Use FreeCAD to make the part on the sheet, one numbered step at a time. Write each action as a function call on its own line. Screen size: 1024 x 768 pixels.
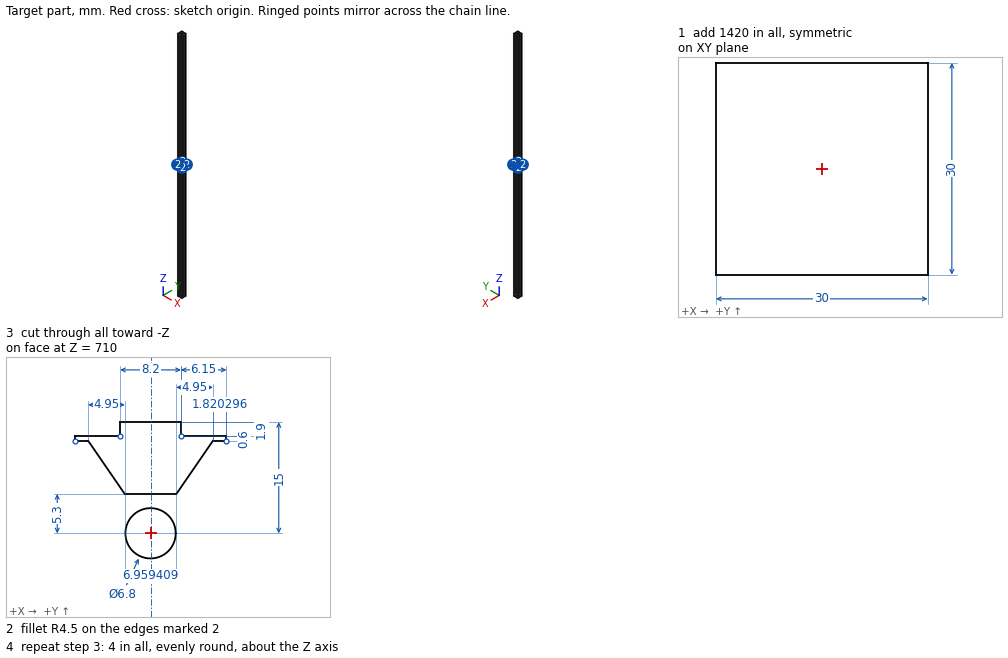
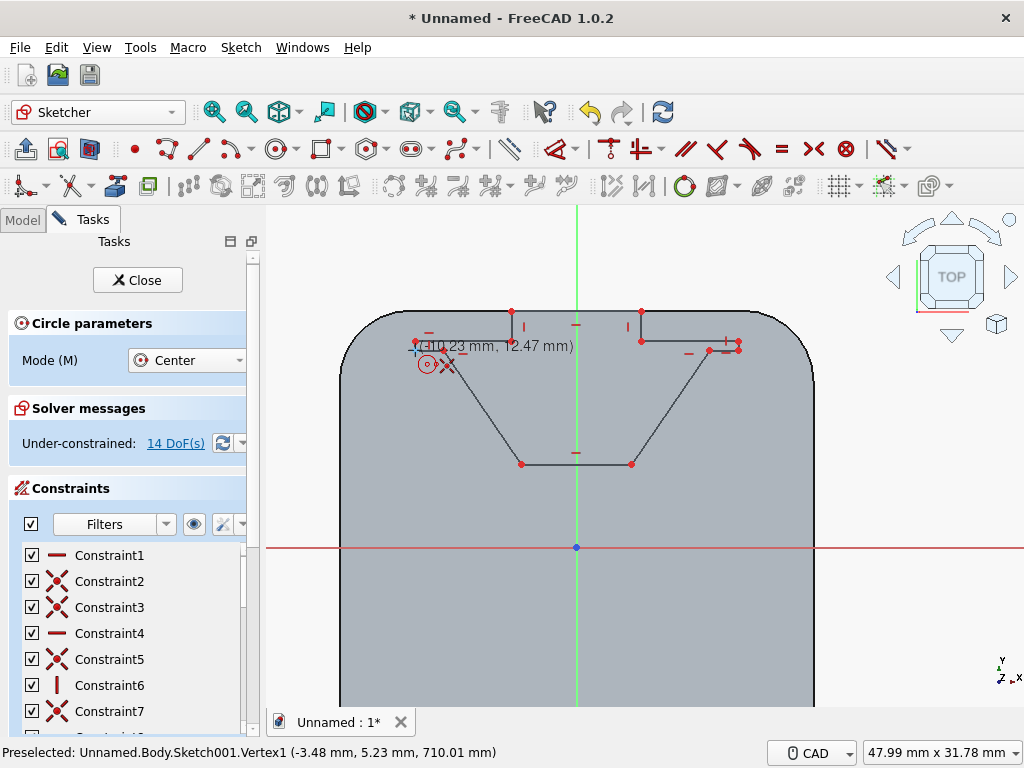
click(577, 548)
click(615, 510)
key(Escape)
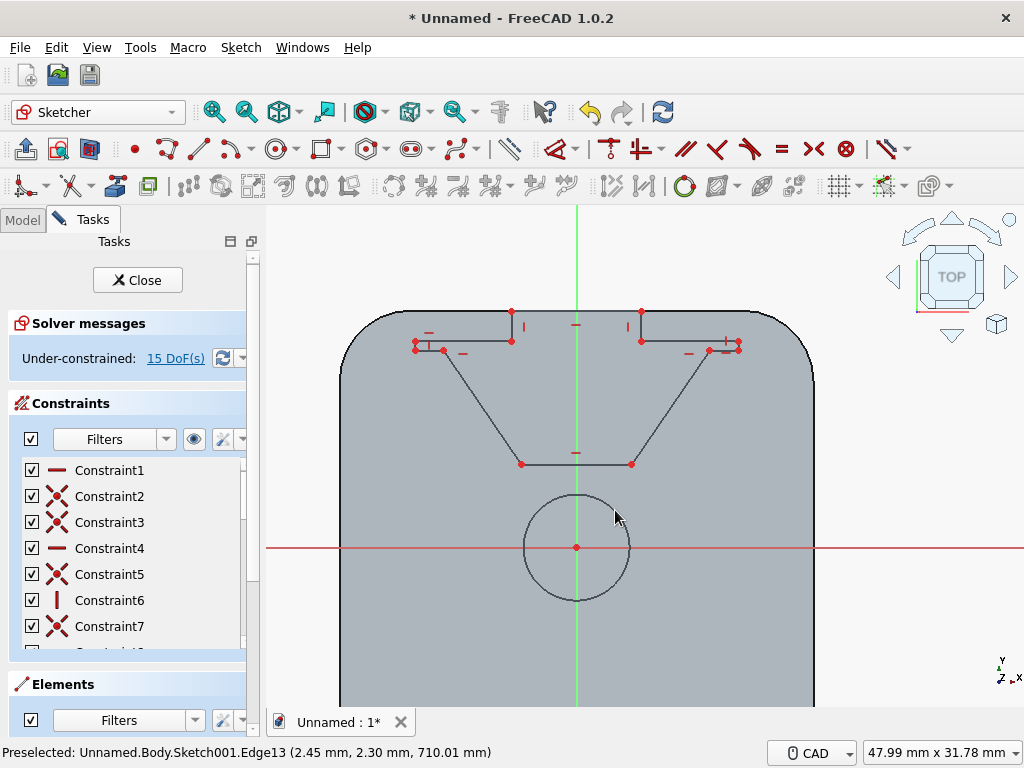
click(641, 341)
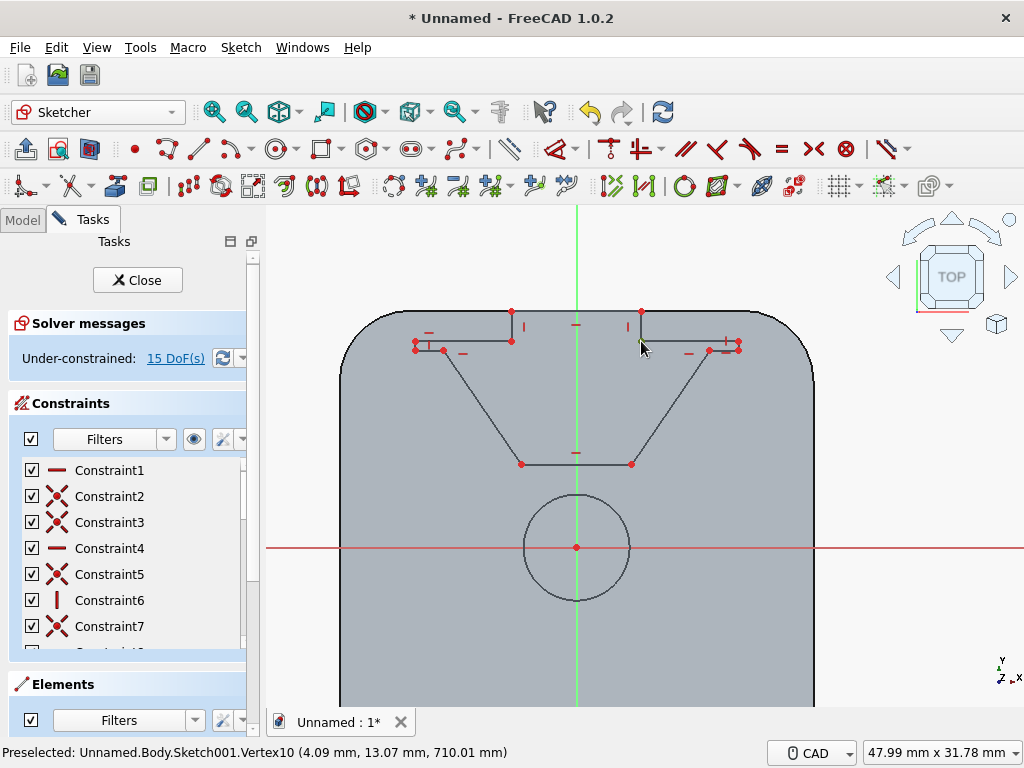
click(512, 341)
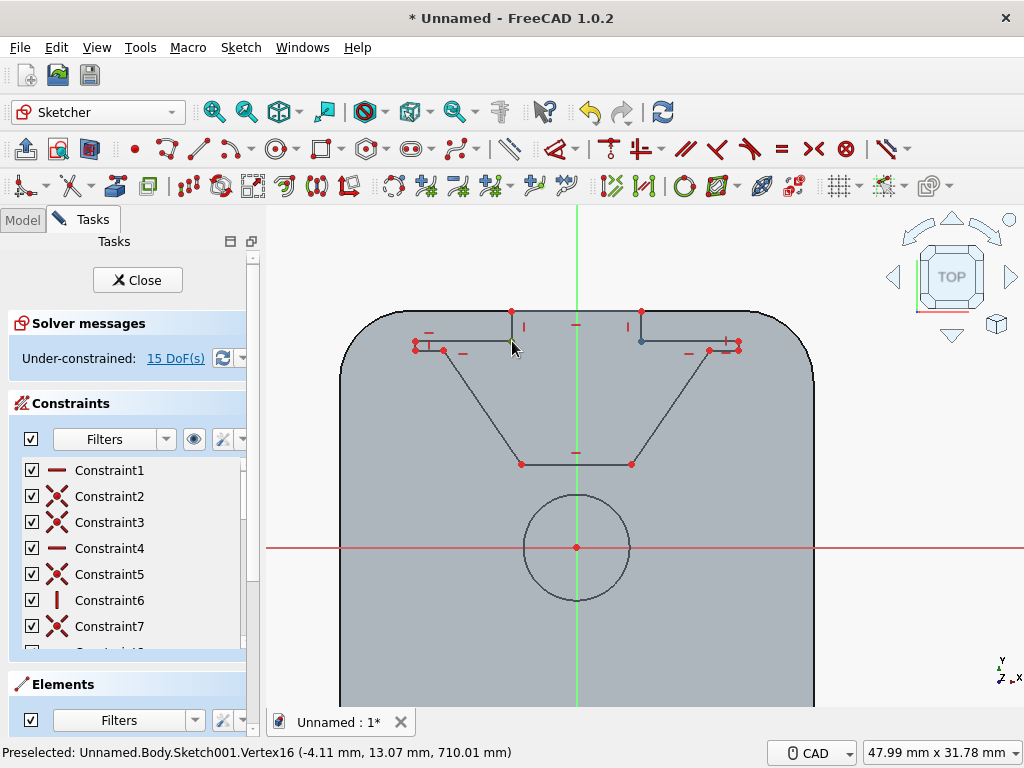
click(577, 647)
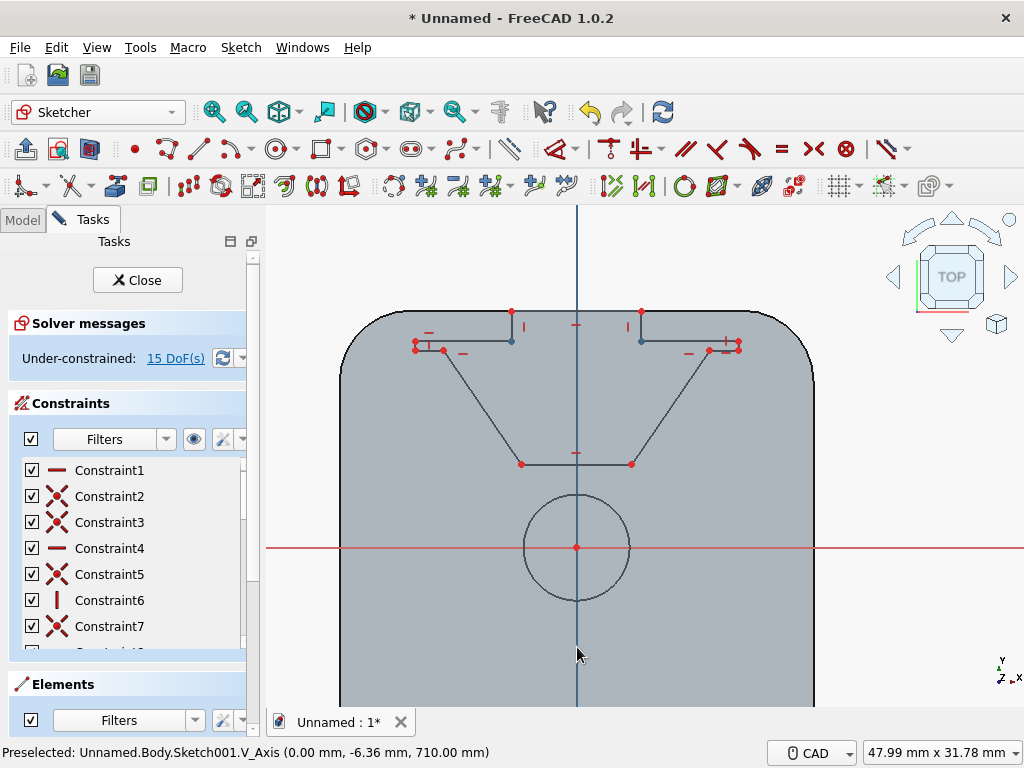
key(s)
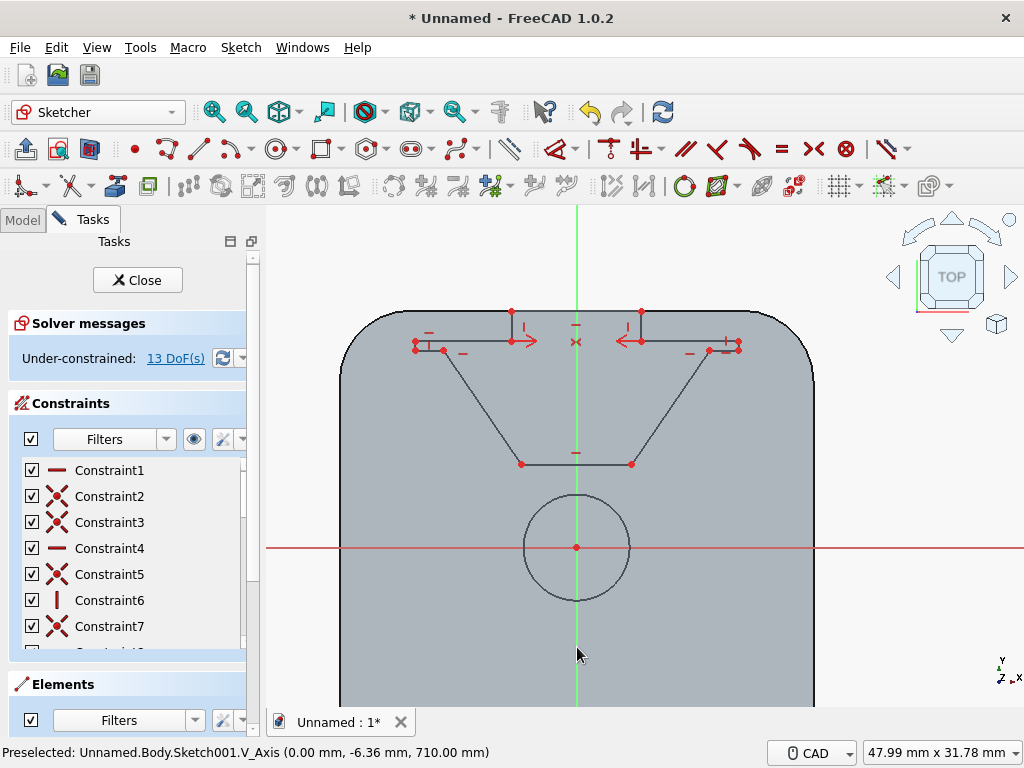
scroll(739, 351, up, 2)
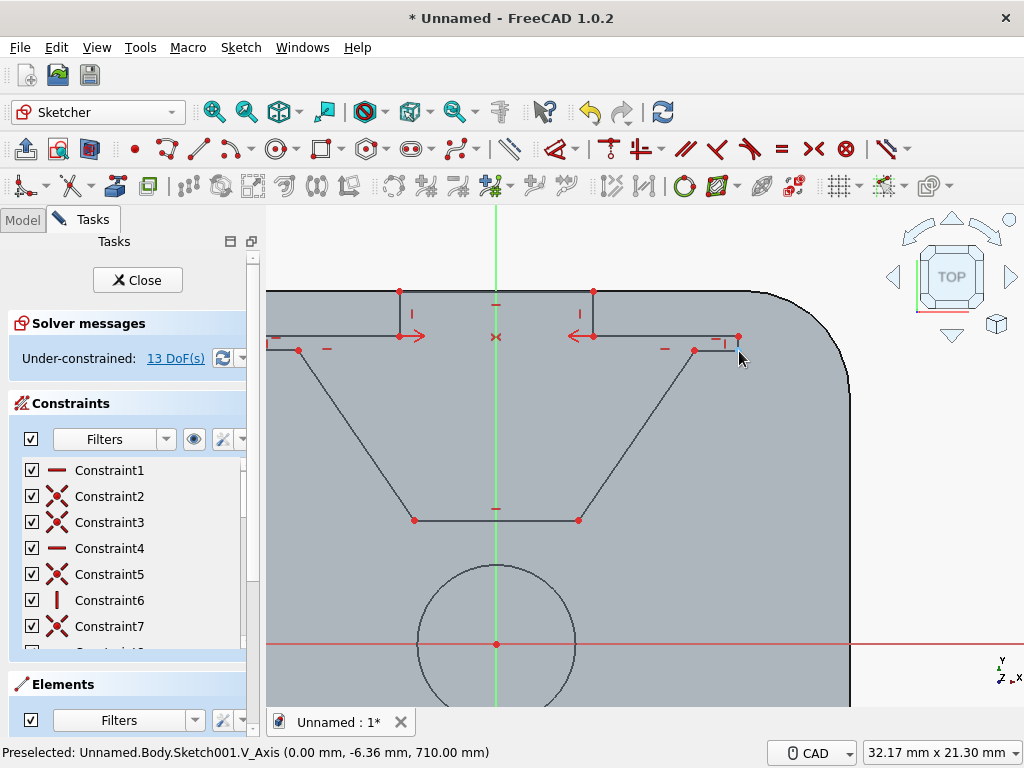
click(738, 351)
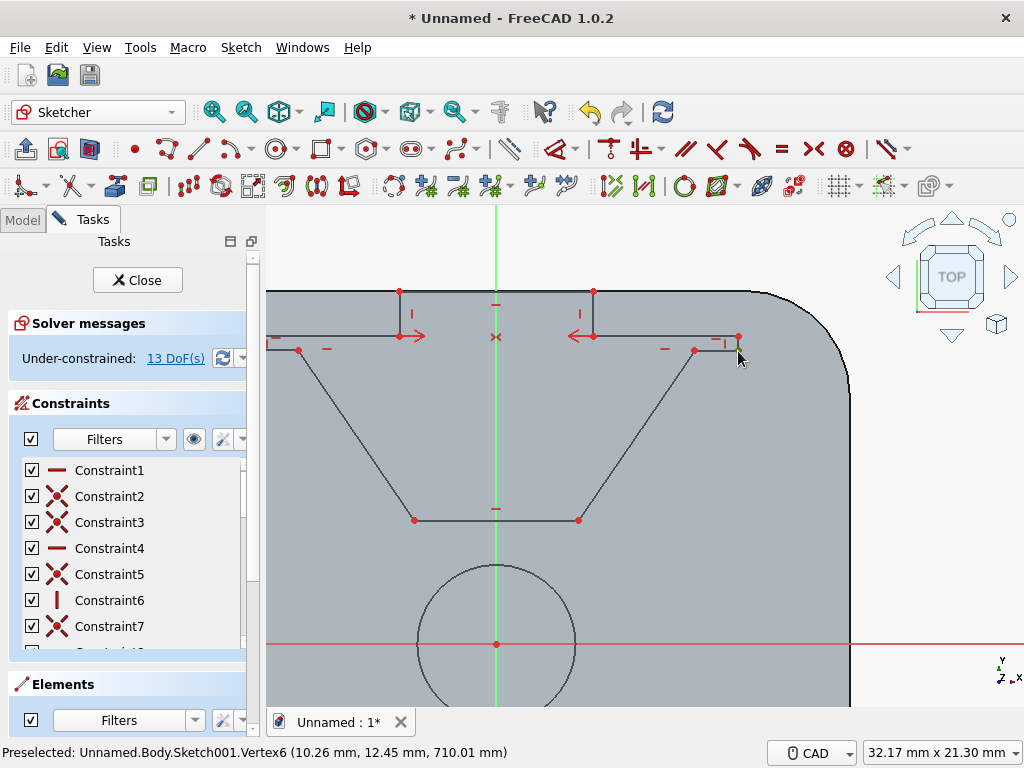
scroll(739, 351, down, 2)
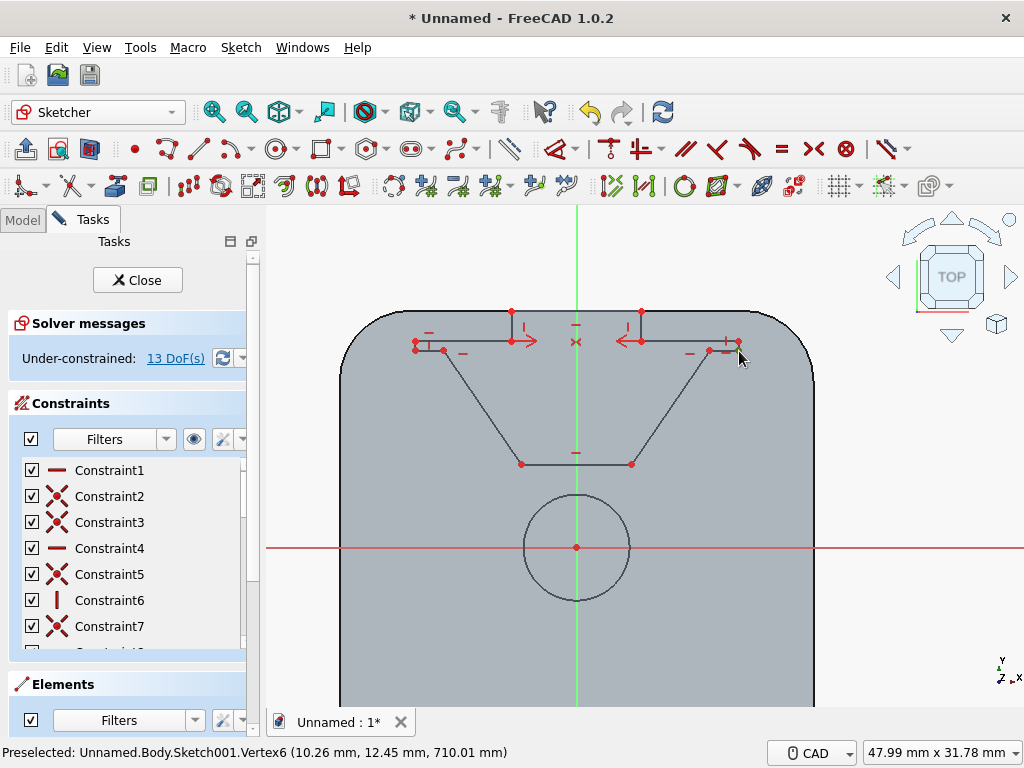
scroll(415, 351, up, 2)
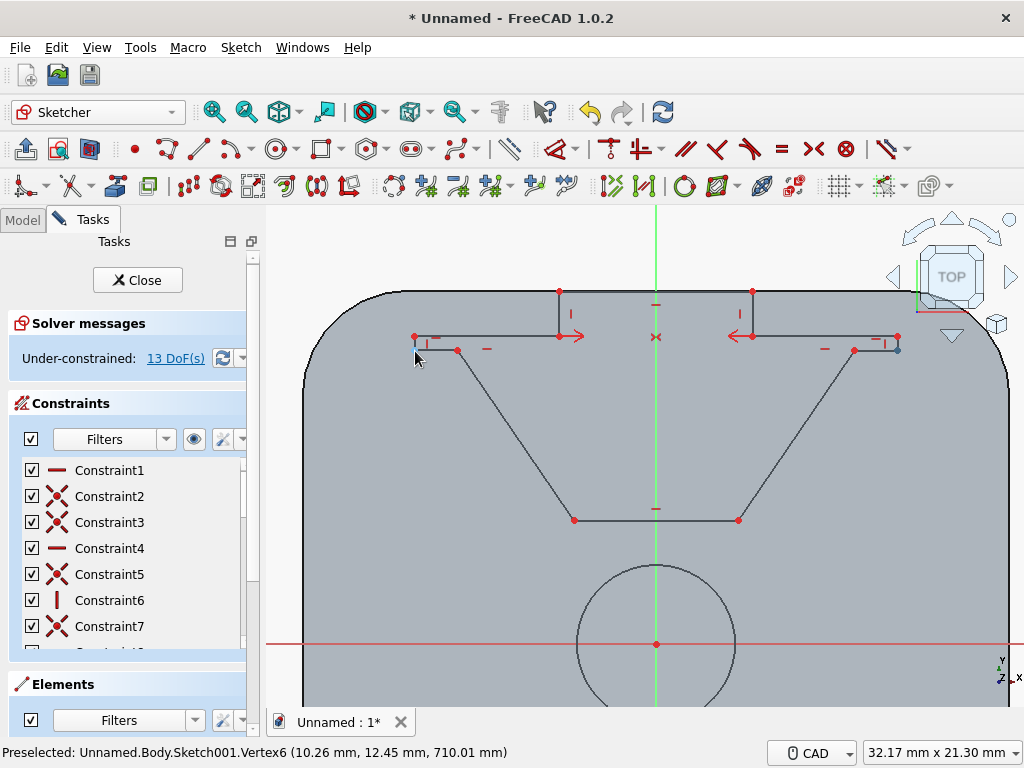
click(415, 350)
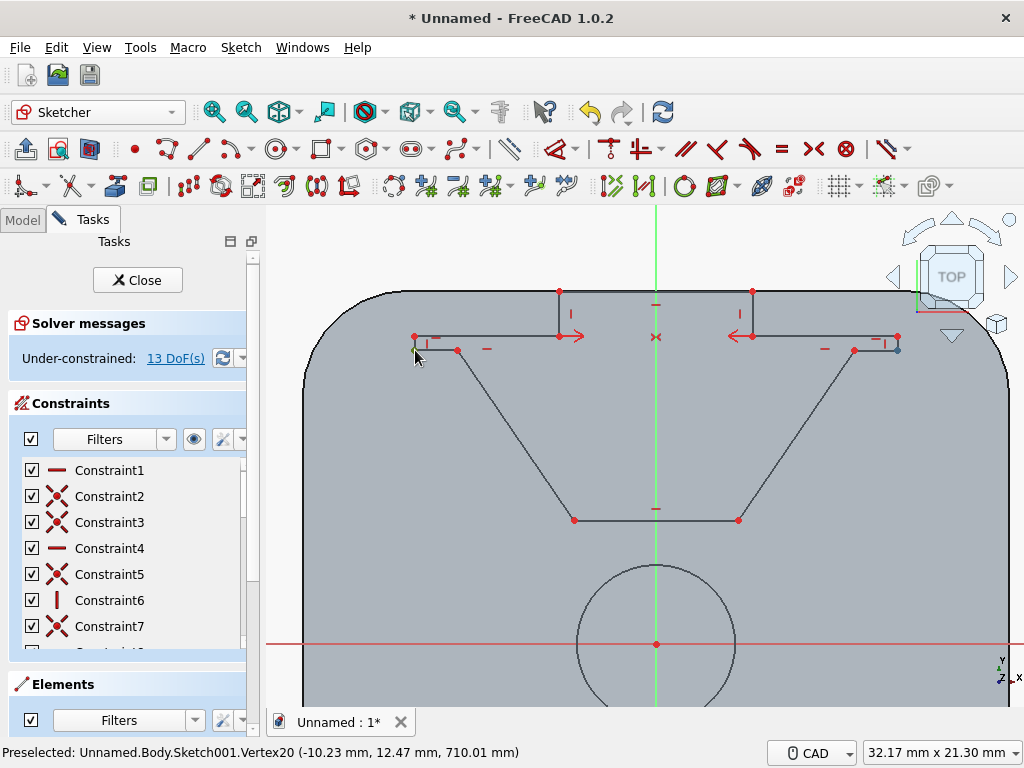
click(656, 488)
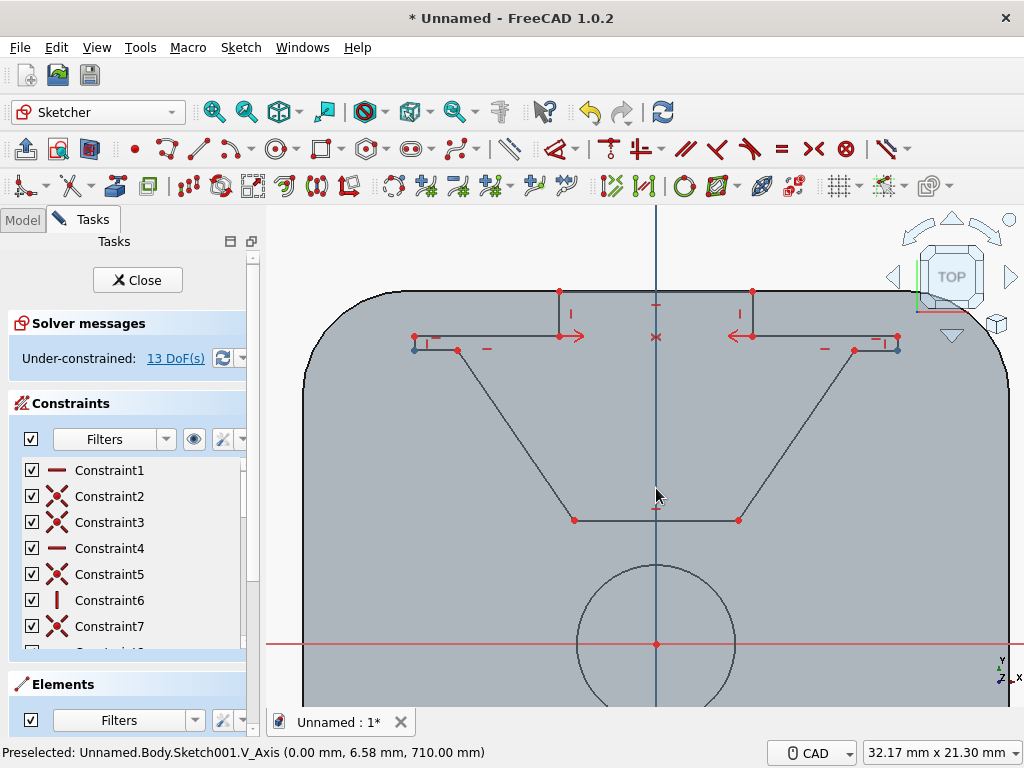
key(s)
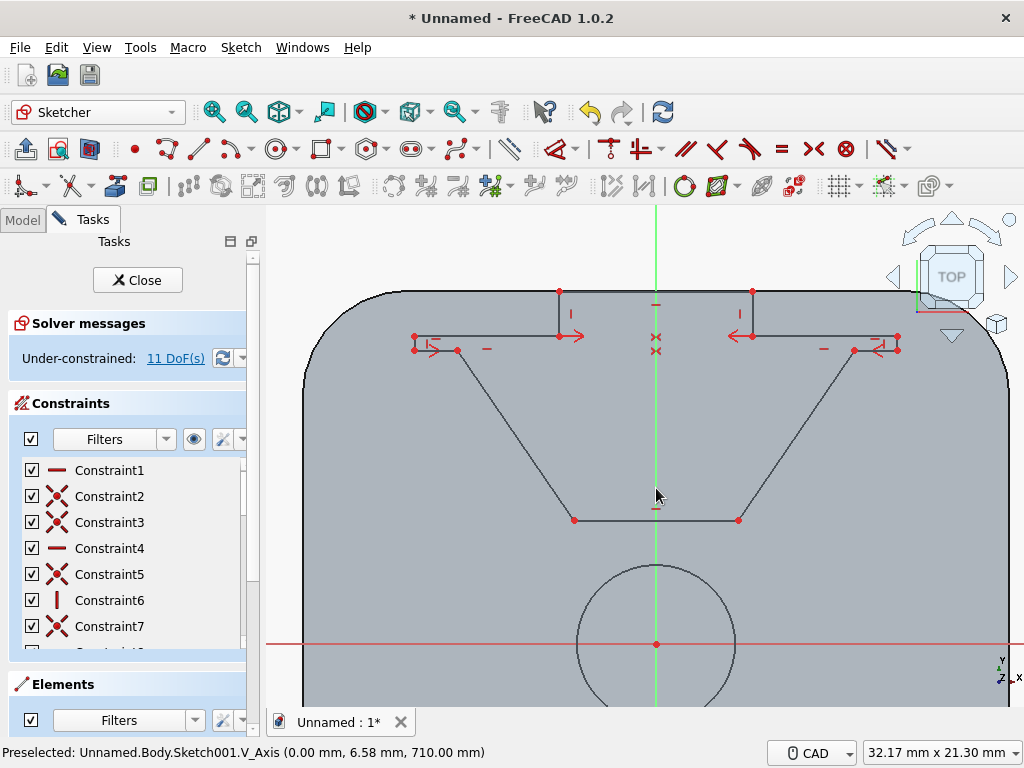
key(d)